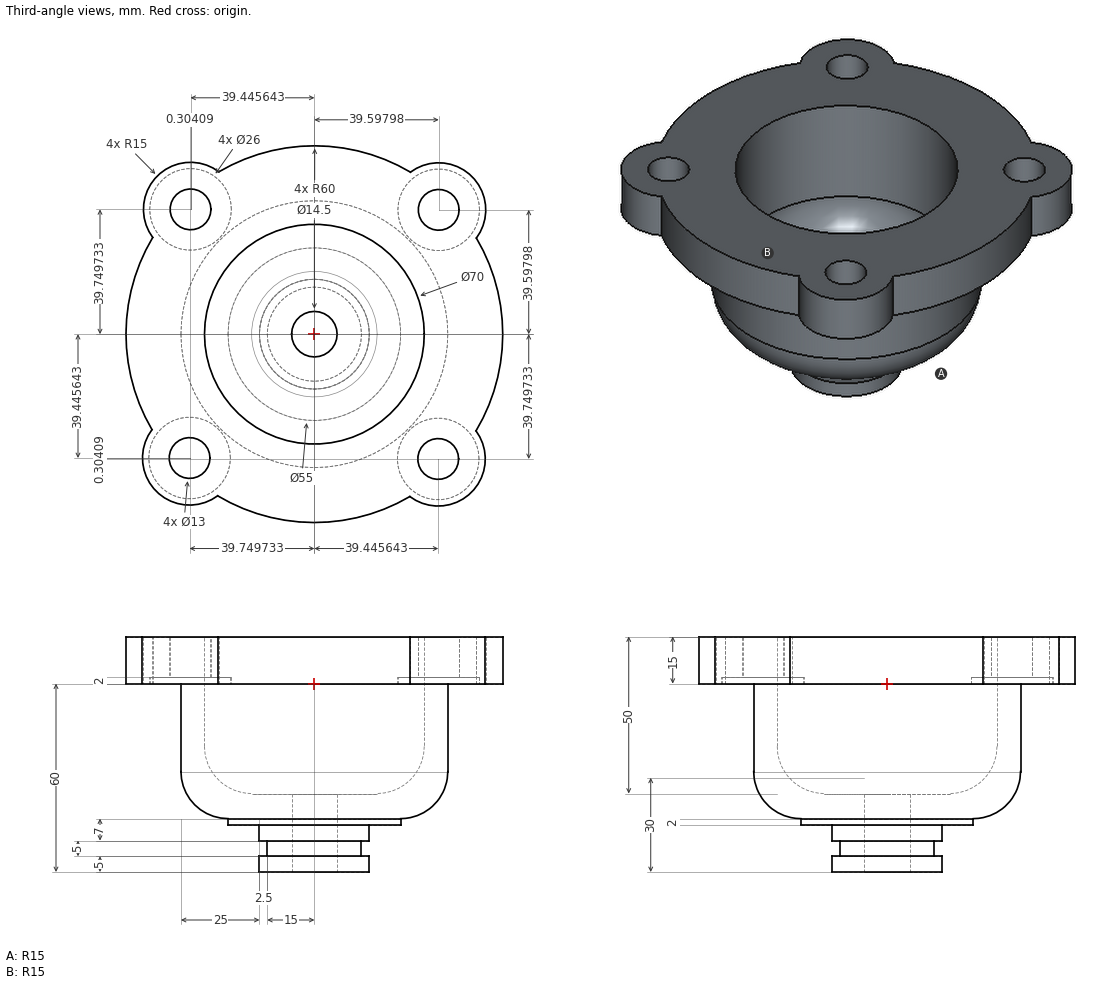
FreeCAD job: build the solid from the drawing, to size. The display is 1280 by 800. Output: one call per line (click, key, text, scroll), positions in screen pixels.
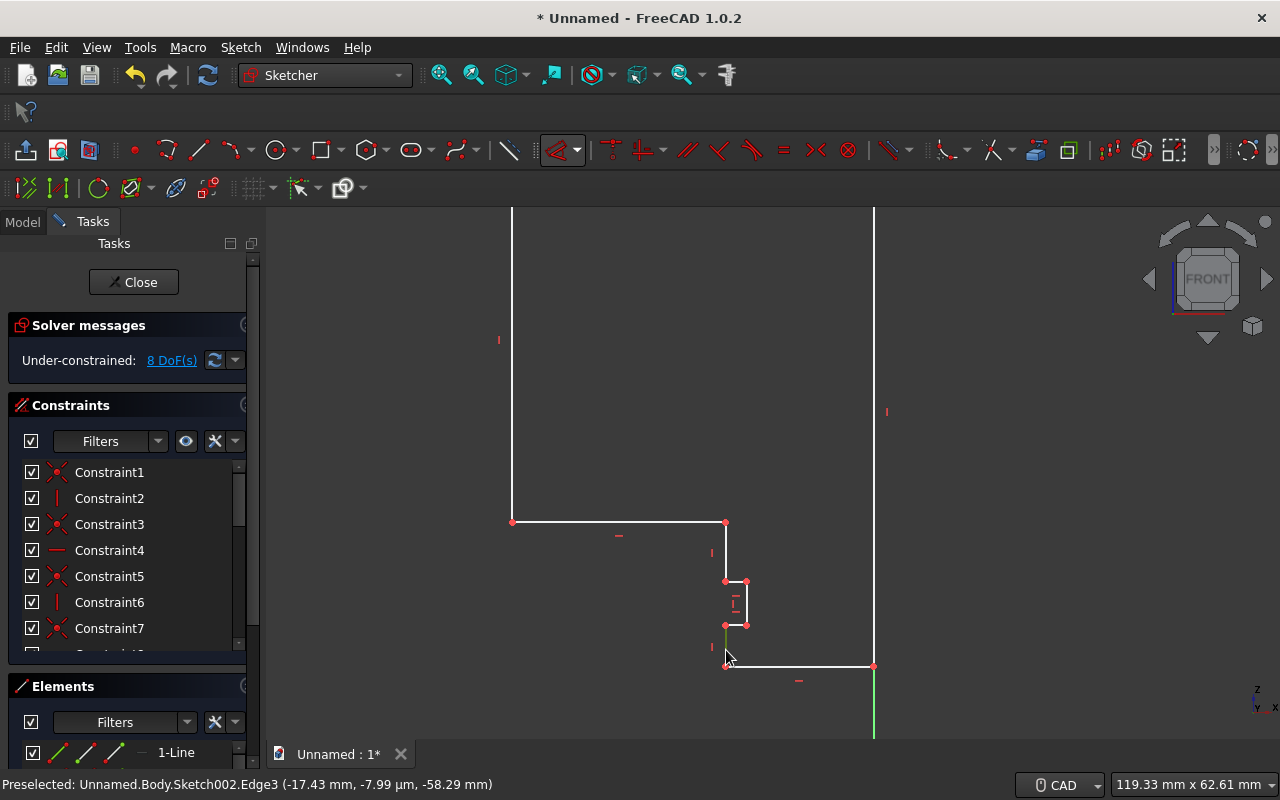
key(i)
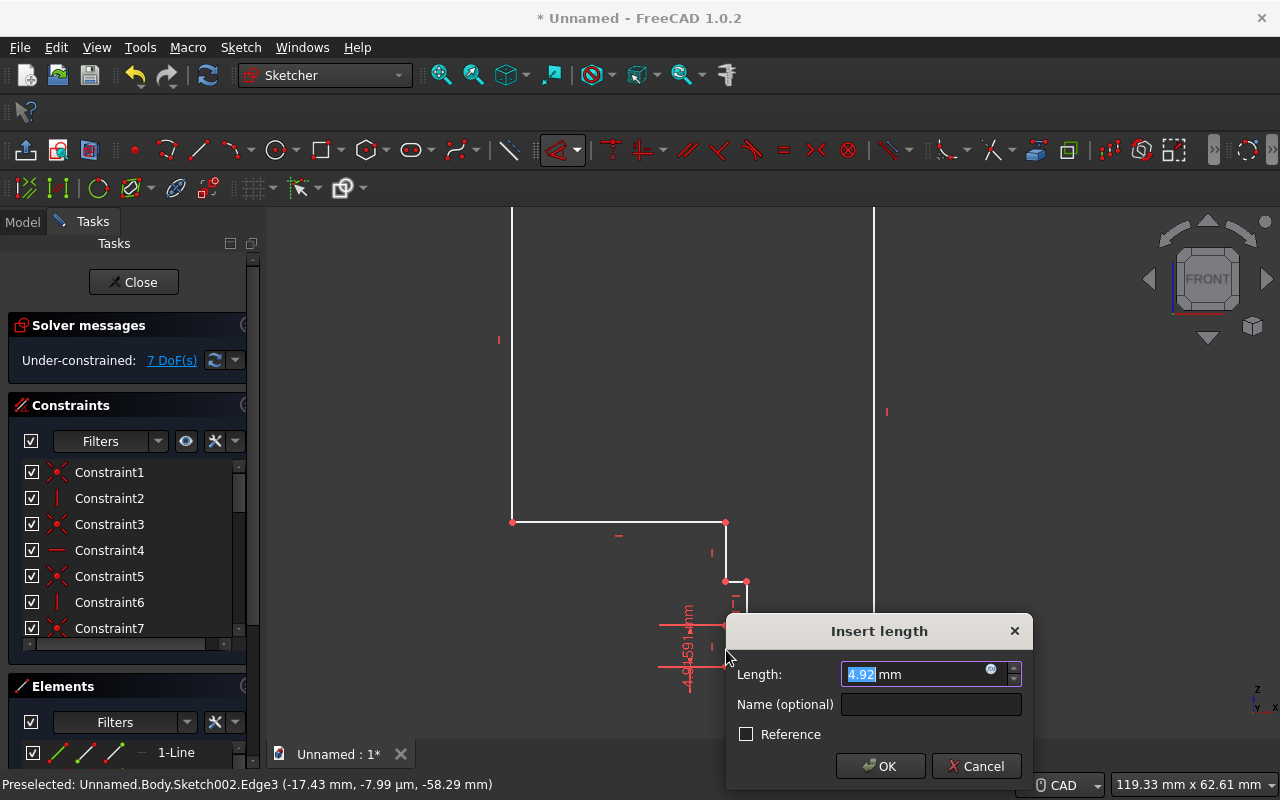
text(5)
key(Return)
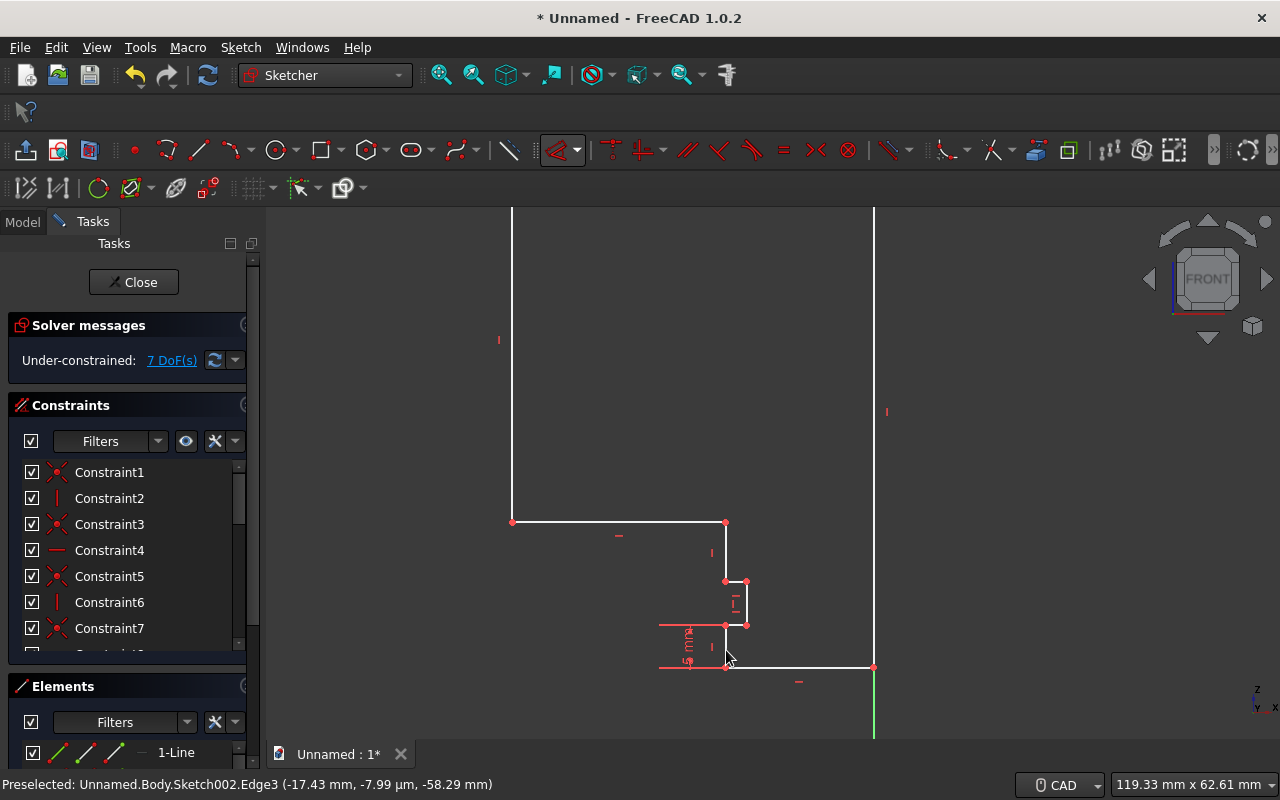
click(747, 612)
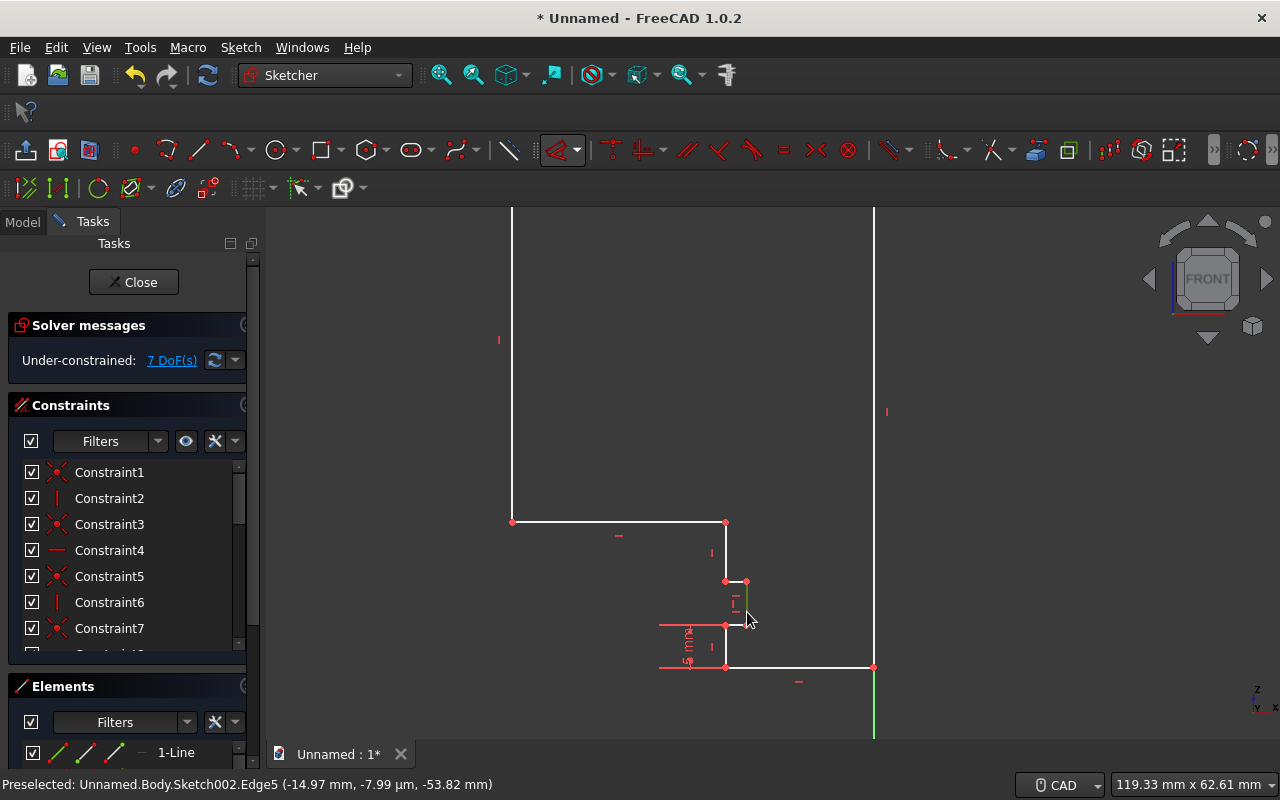
key(i)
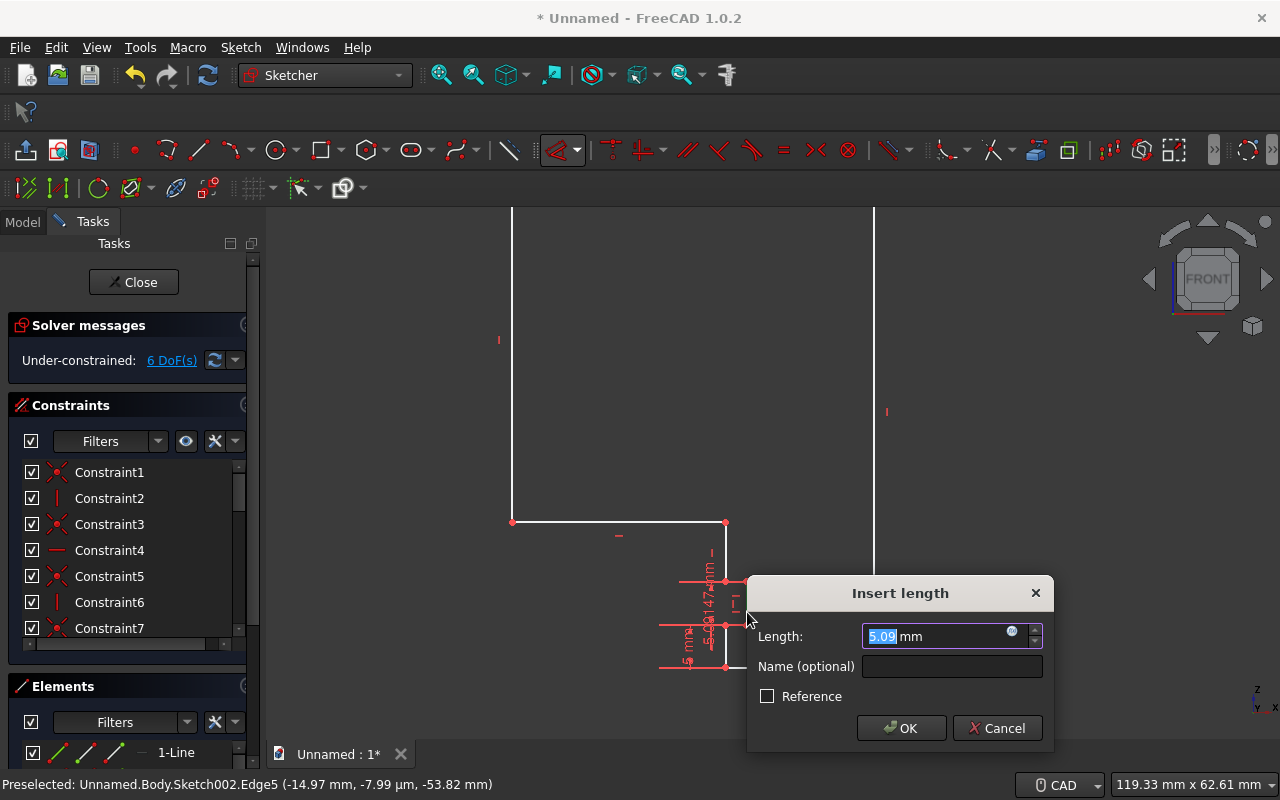
text(5)
key(Return)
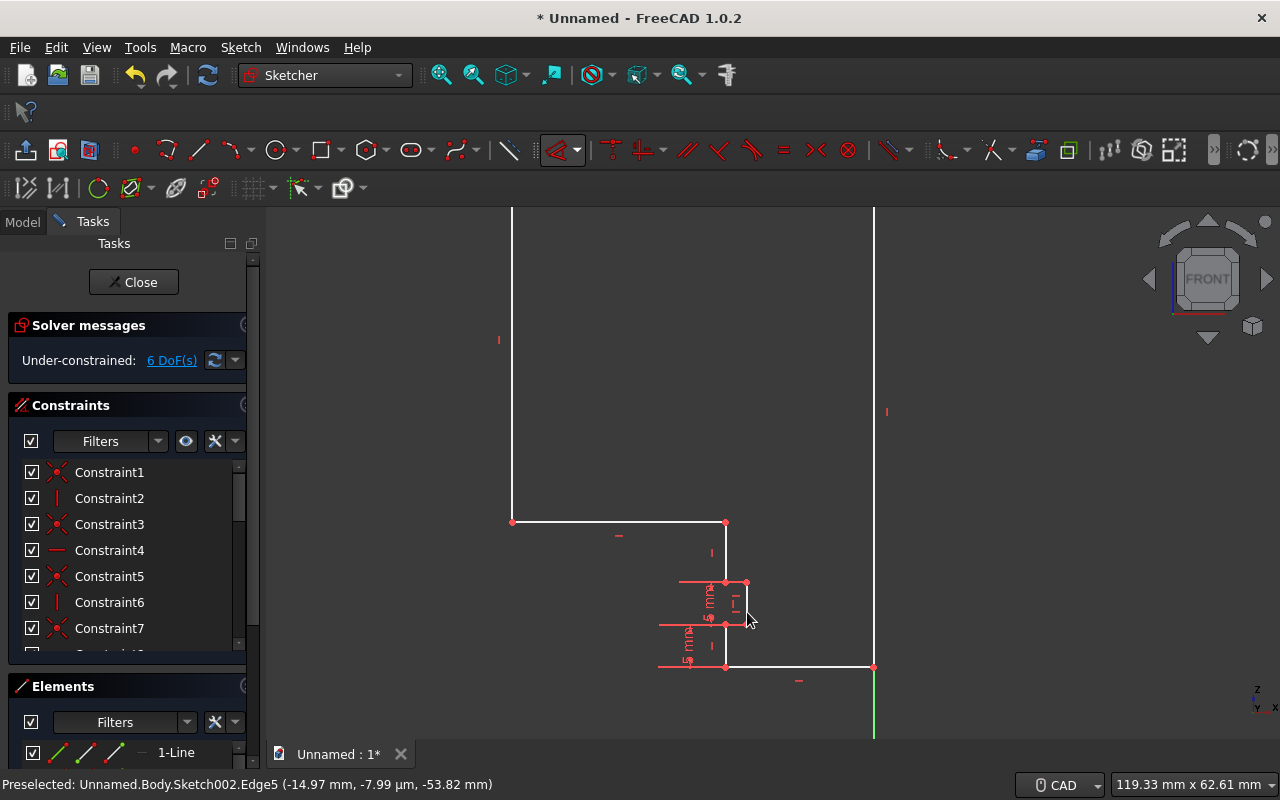
click(726, 564)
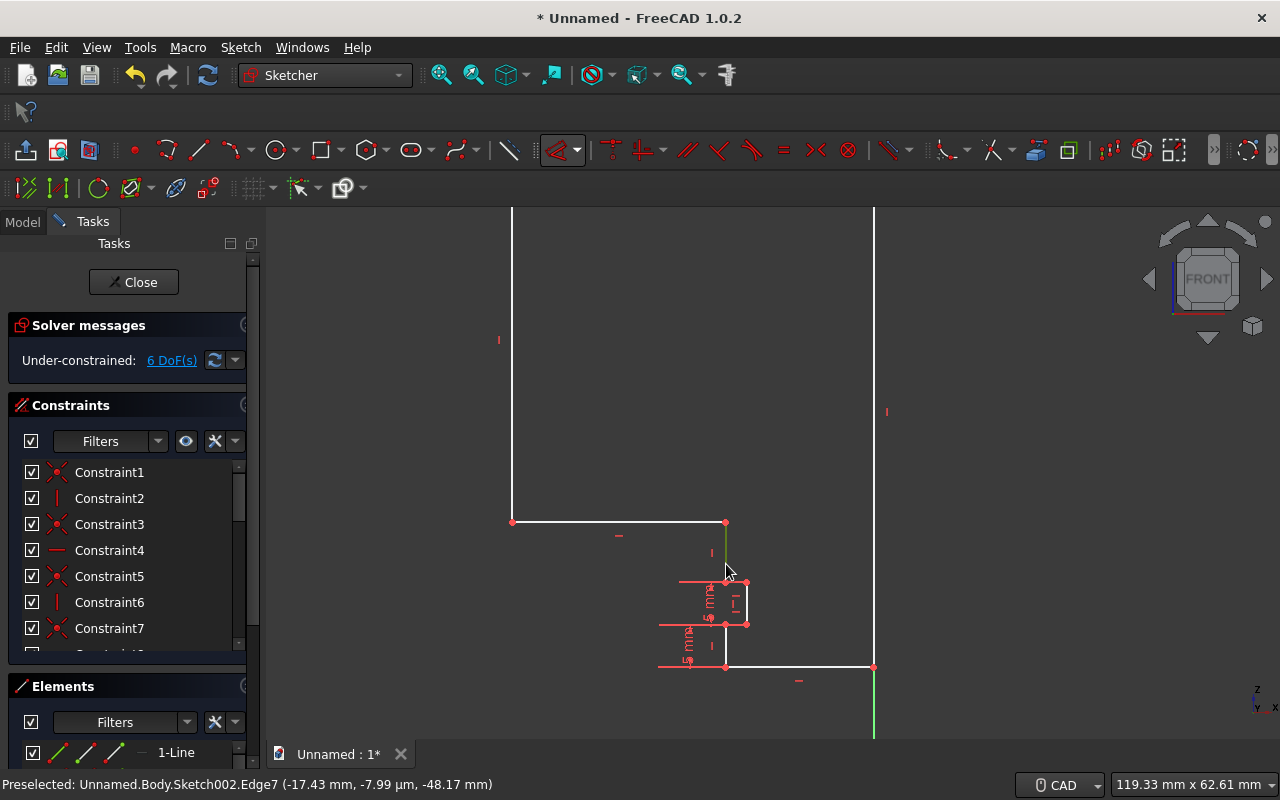
click(580, 150)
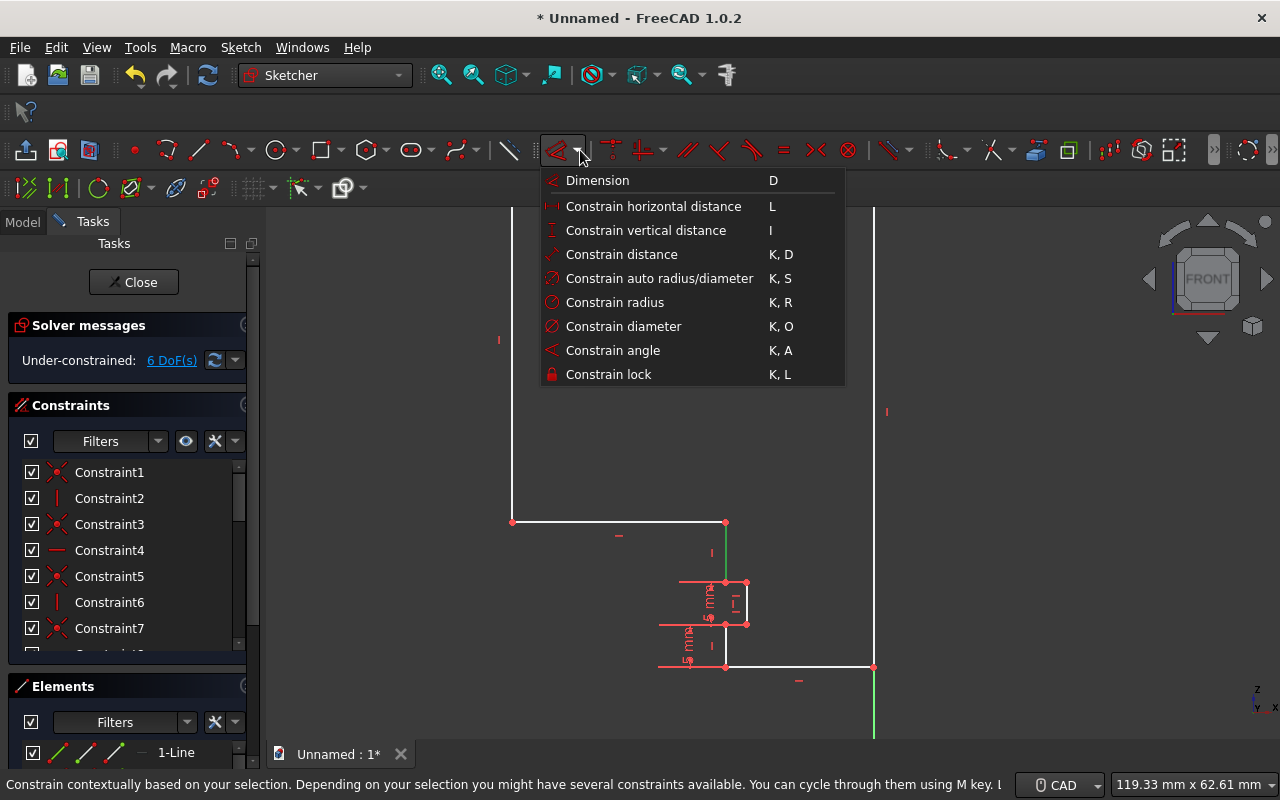
click(693, 230)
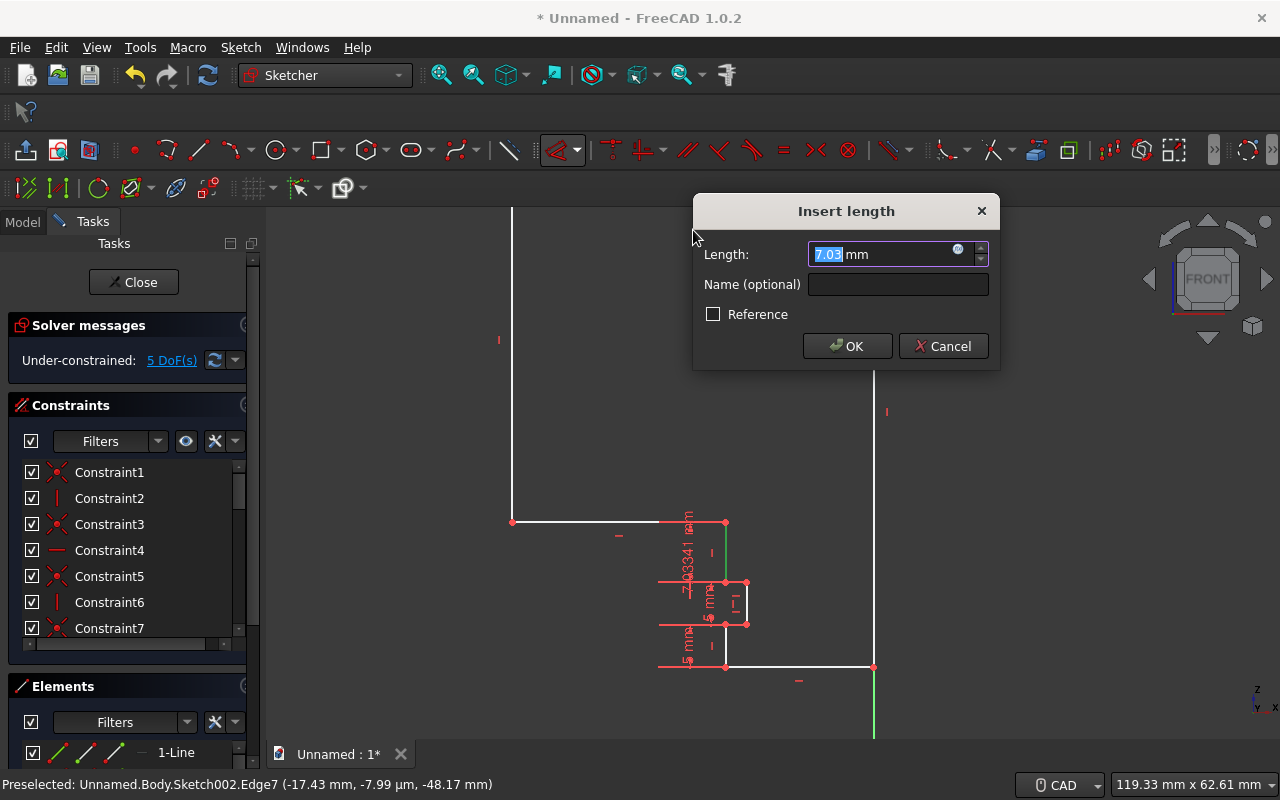
text(7)
key(Return)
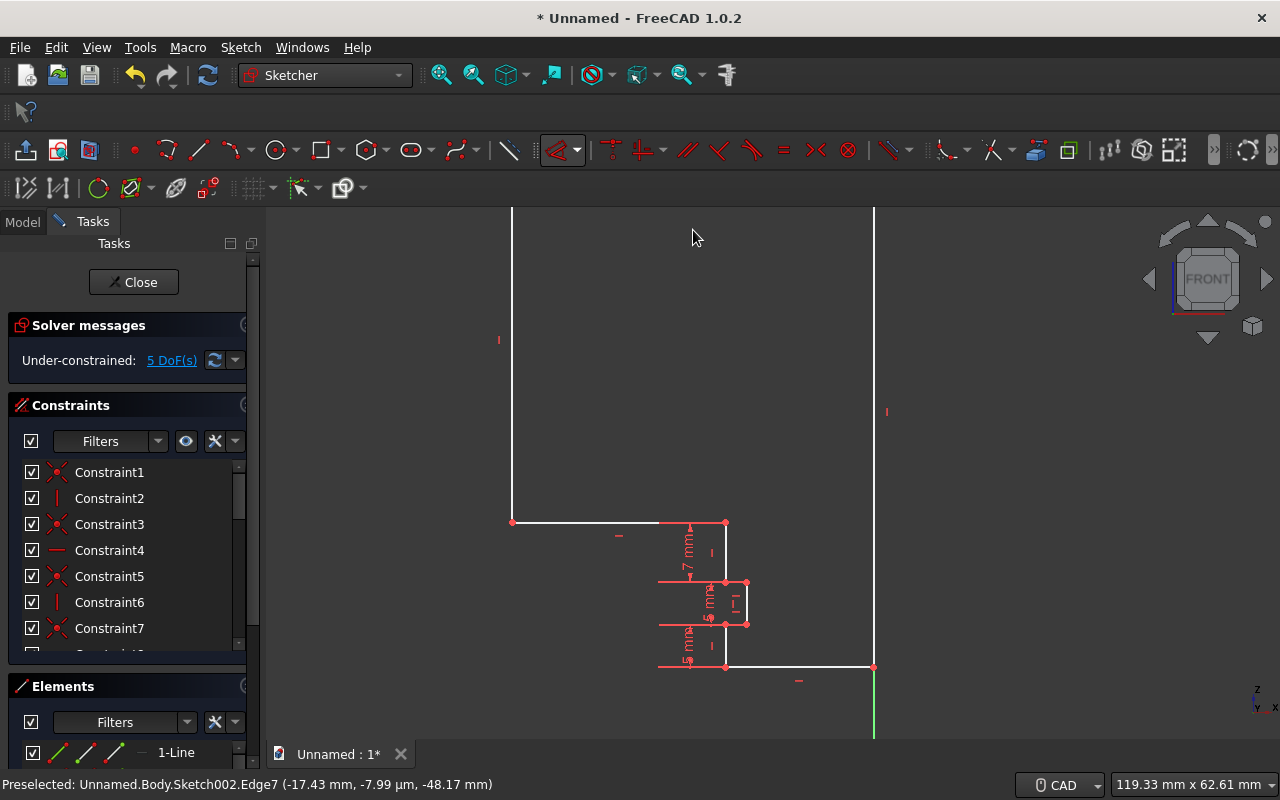
click(874, 309)